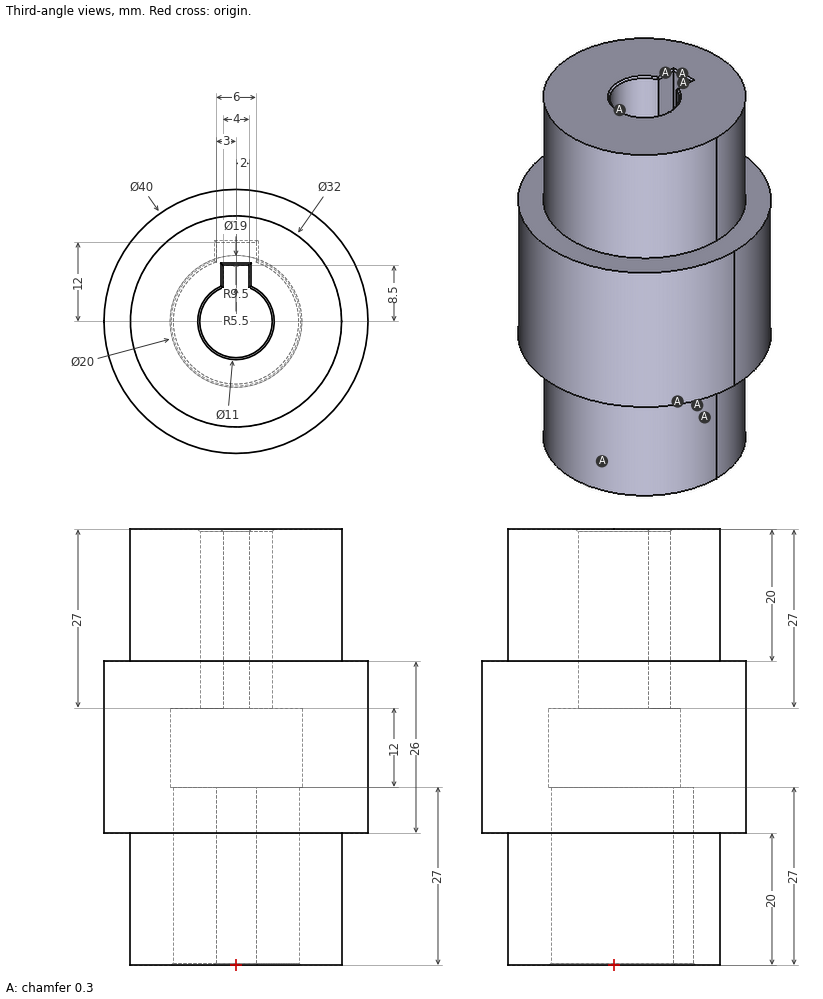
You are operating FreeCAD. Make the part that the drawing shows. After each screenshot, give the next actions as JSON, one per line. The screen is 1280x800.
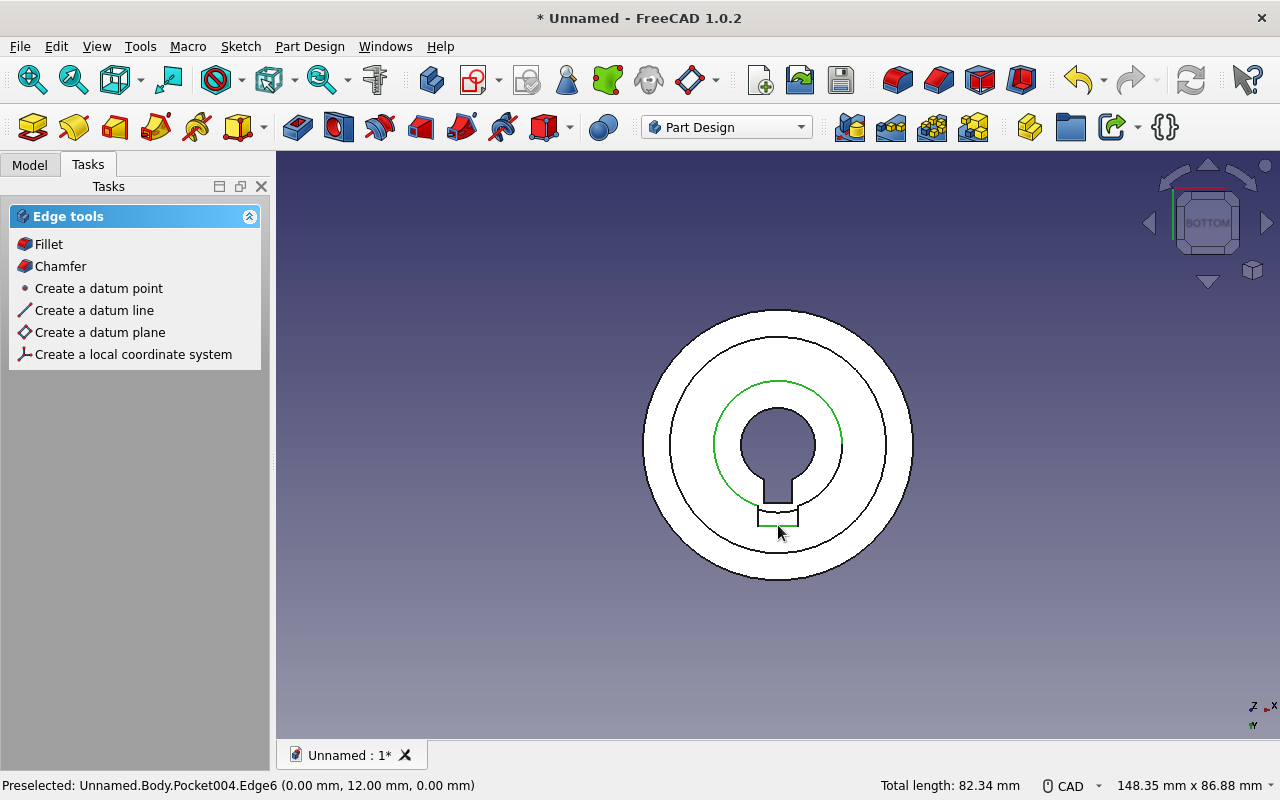
{"action": "left_click", "coordinate": [798, 515], "text": "ctrl"}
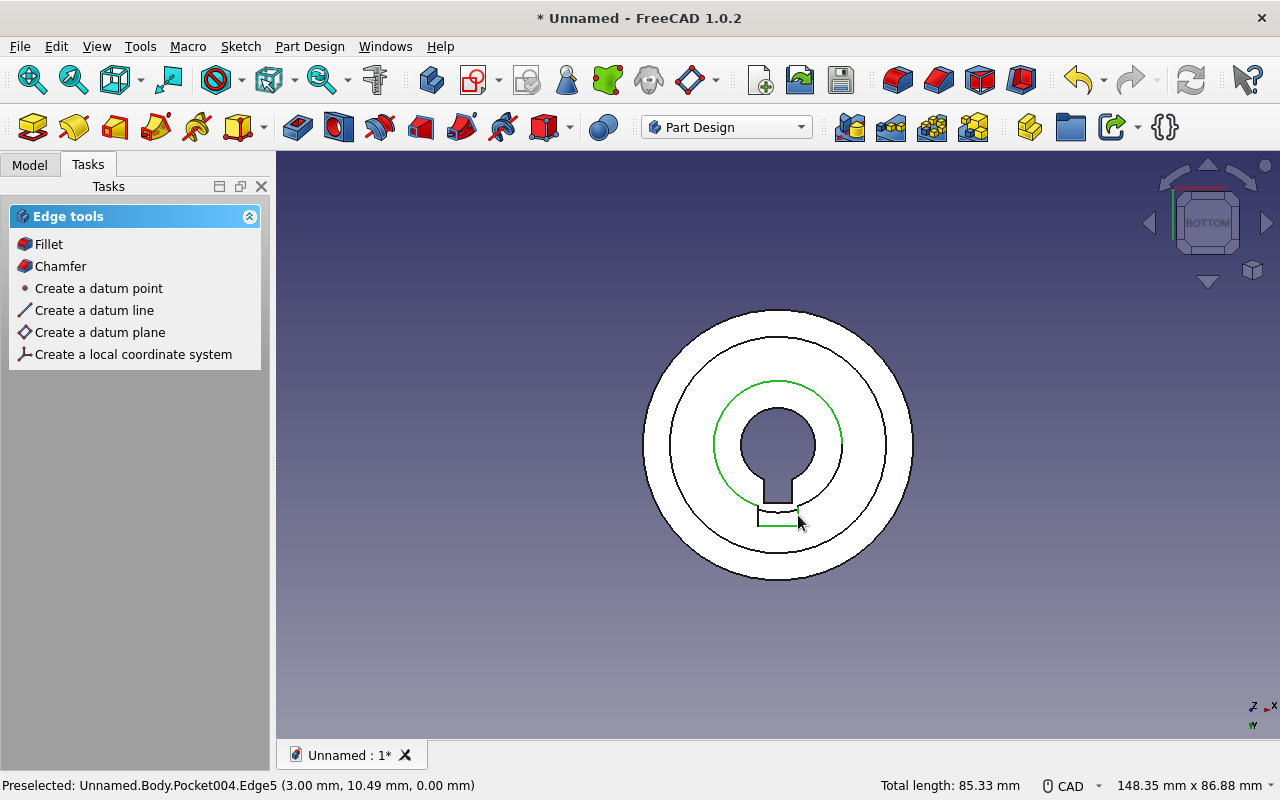
{"action": "left_click", "coordinate": [758, 515], "text": "ctrl"}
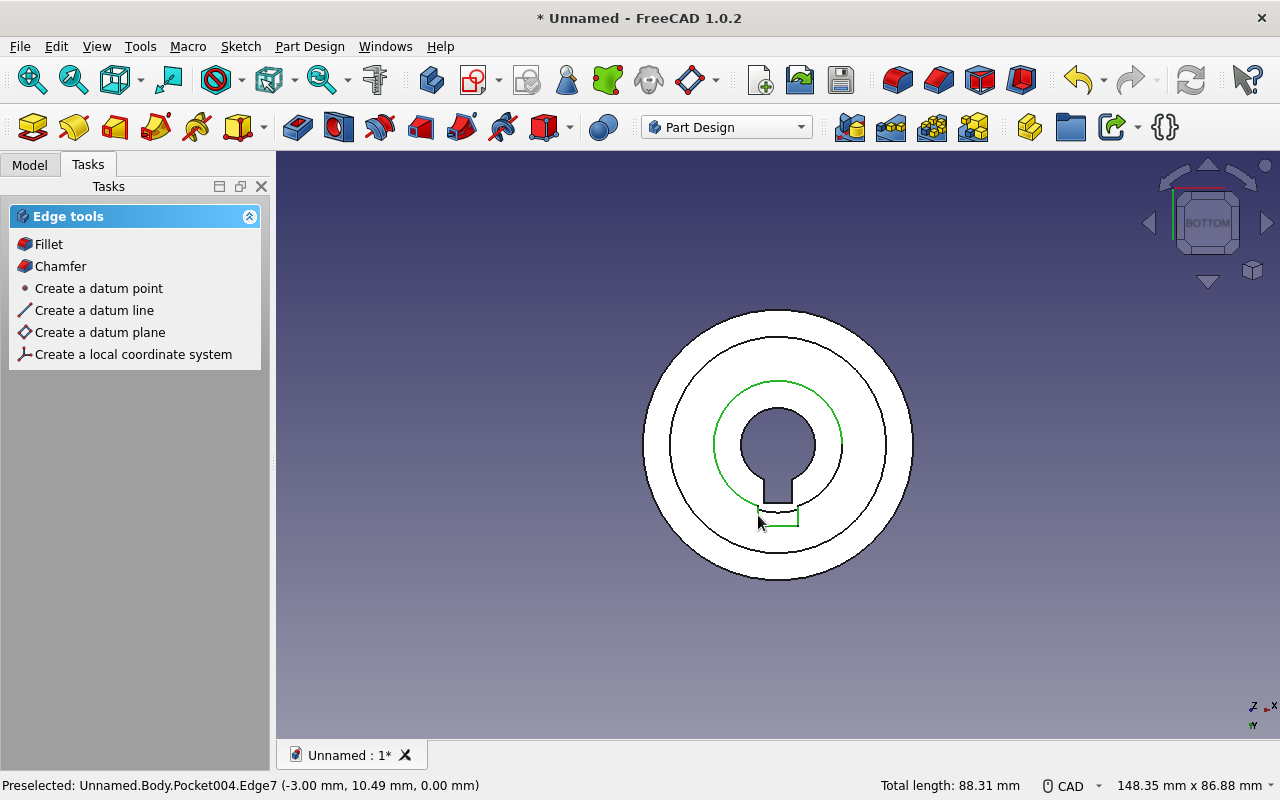
{"action": "left_click", "coordinate": [939, 80]}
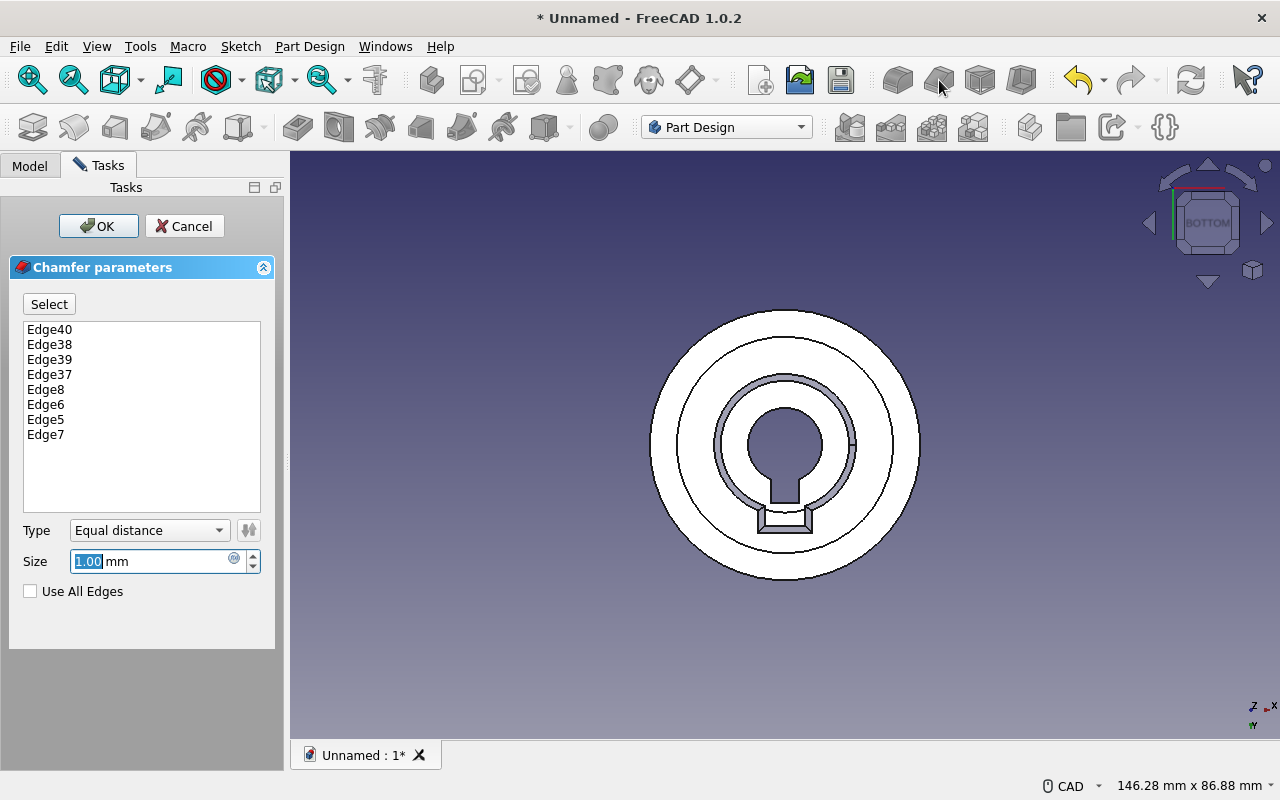
{"action": "type", "text": "0.3"}
{"action": "key", "text": "Tab"}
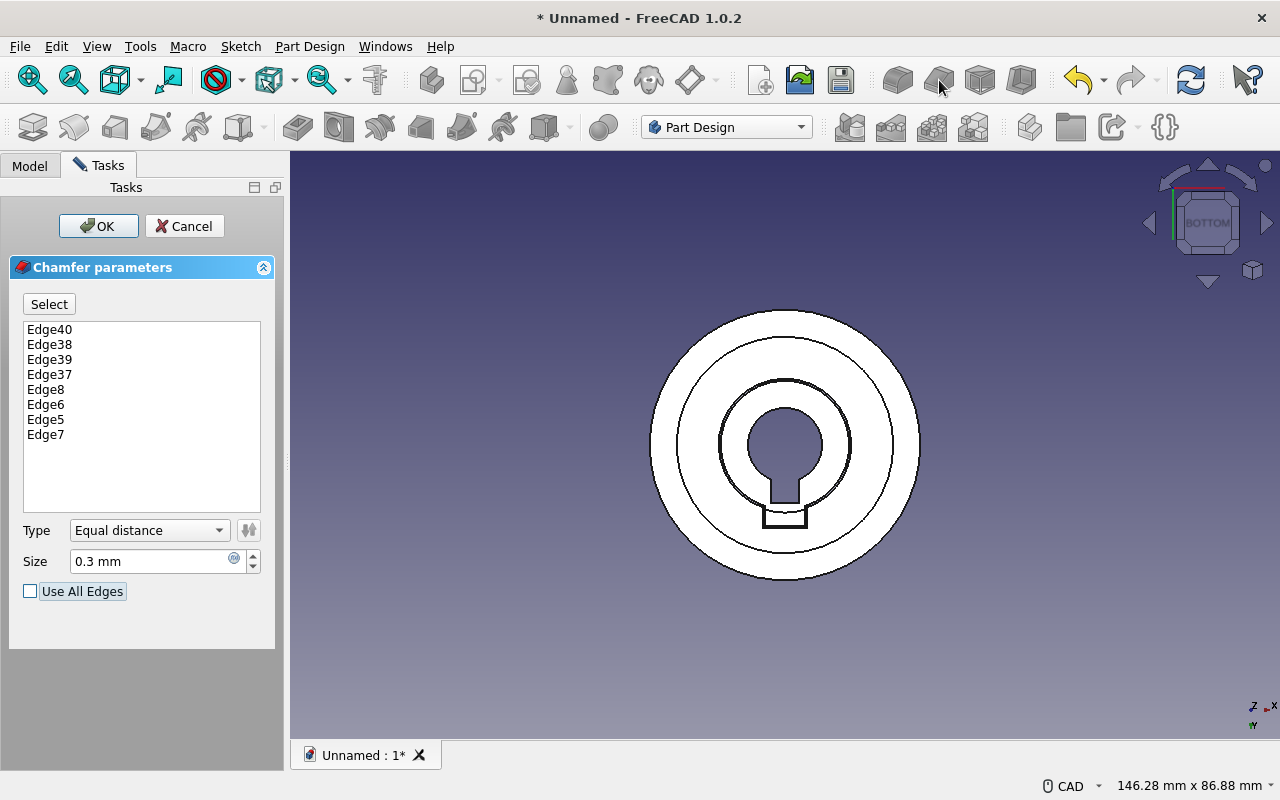
{"action": "left_click", "coordinate": [99, 226]}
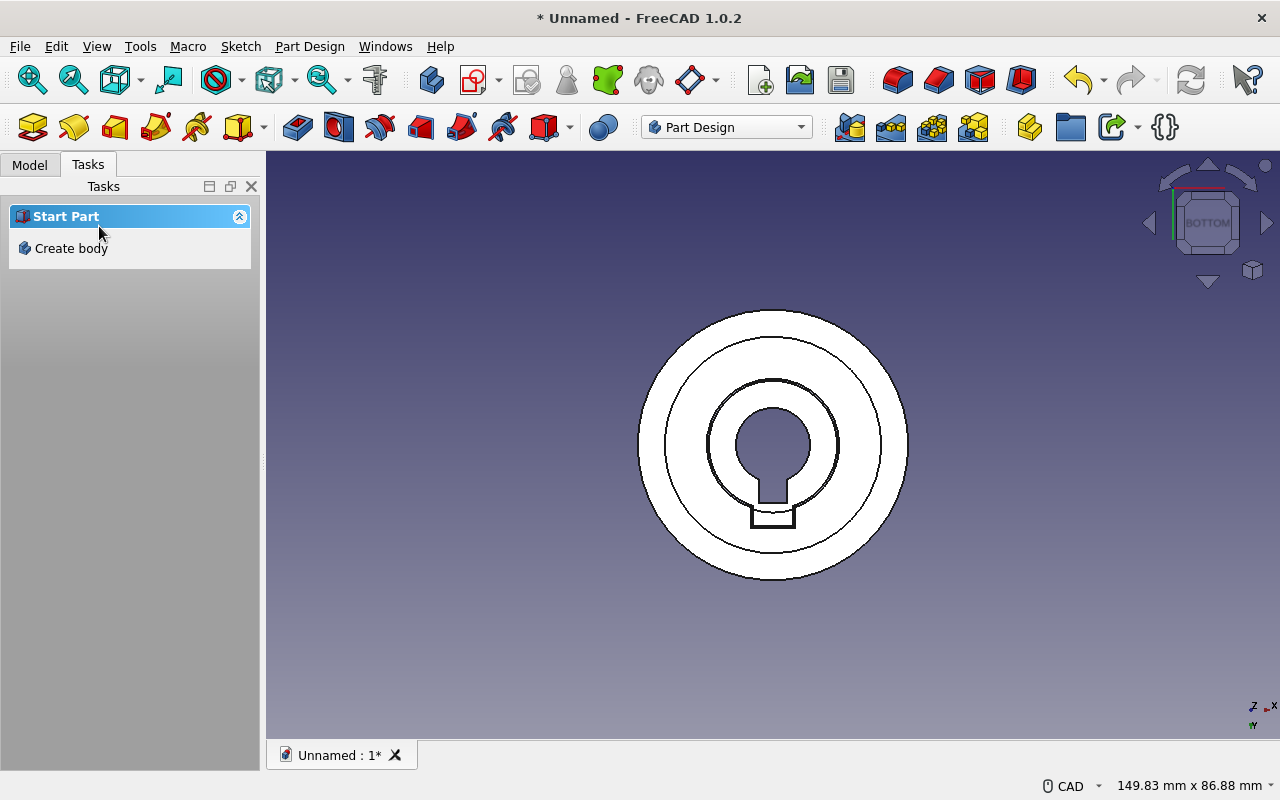
{"action": "key", "text": "0"}